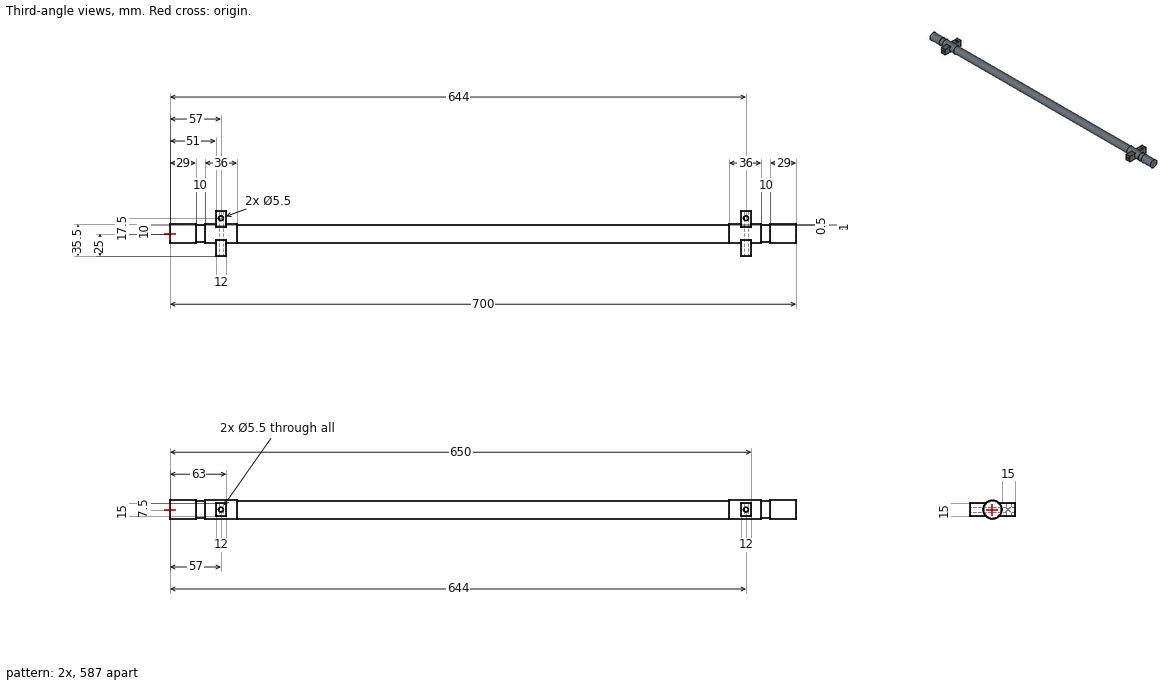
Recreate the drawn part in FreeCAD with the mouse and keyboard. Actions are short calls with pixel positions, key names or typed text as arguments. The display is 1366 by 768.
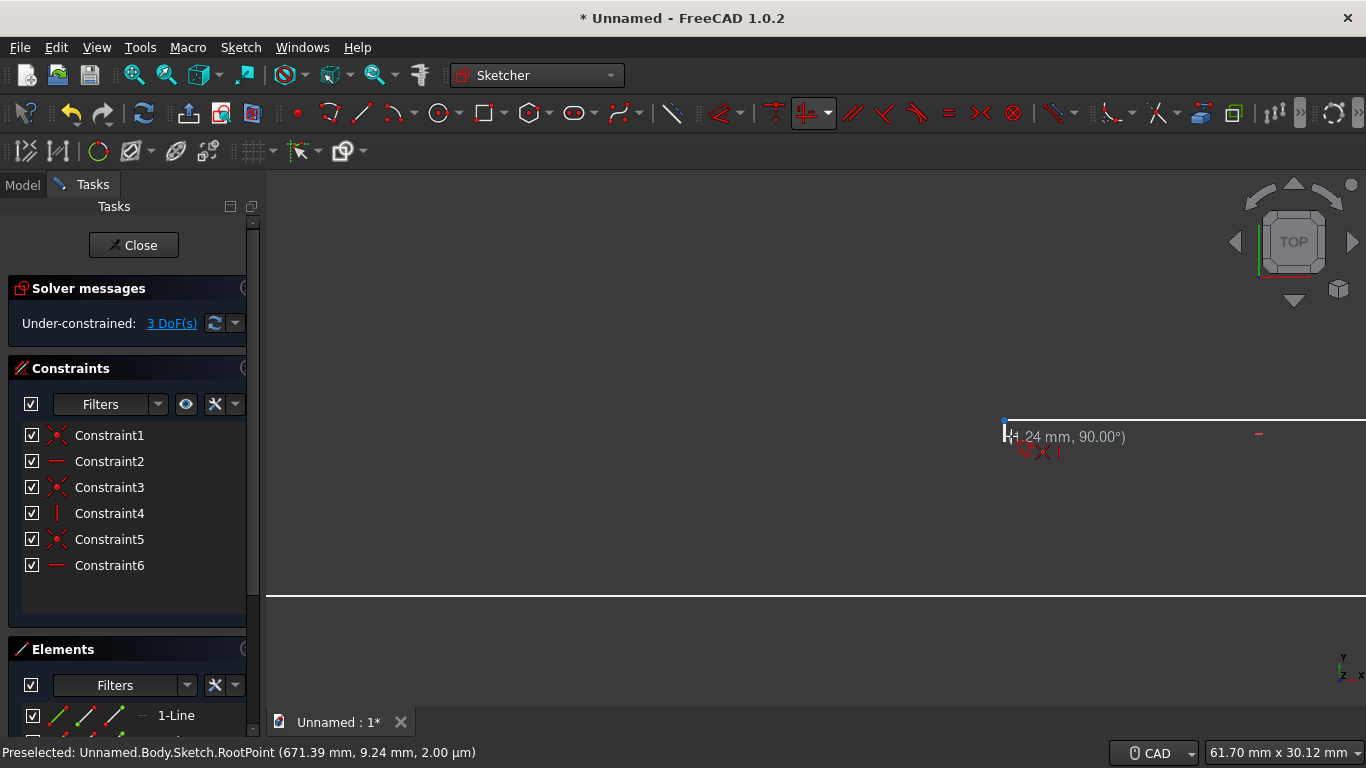
click(1004, 426)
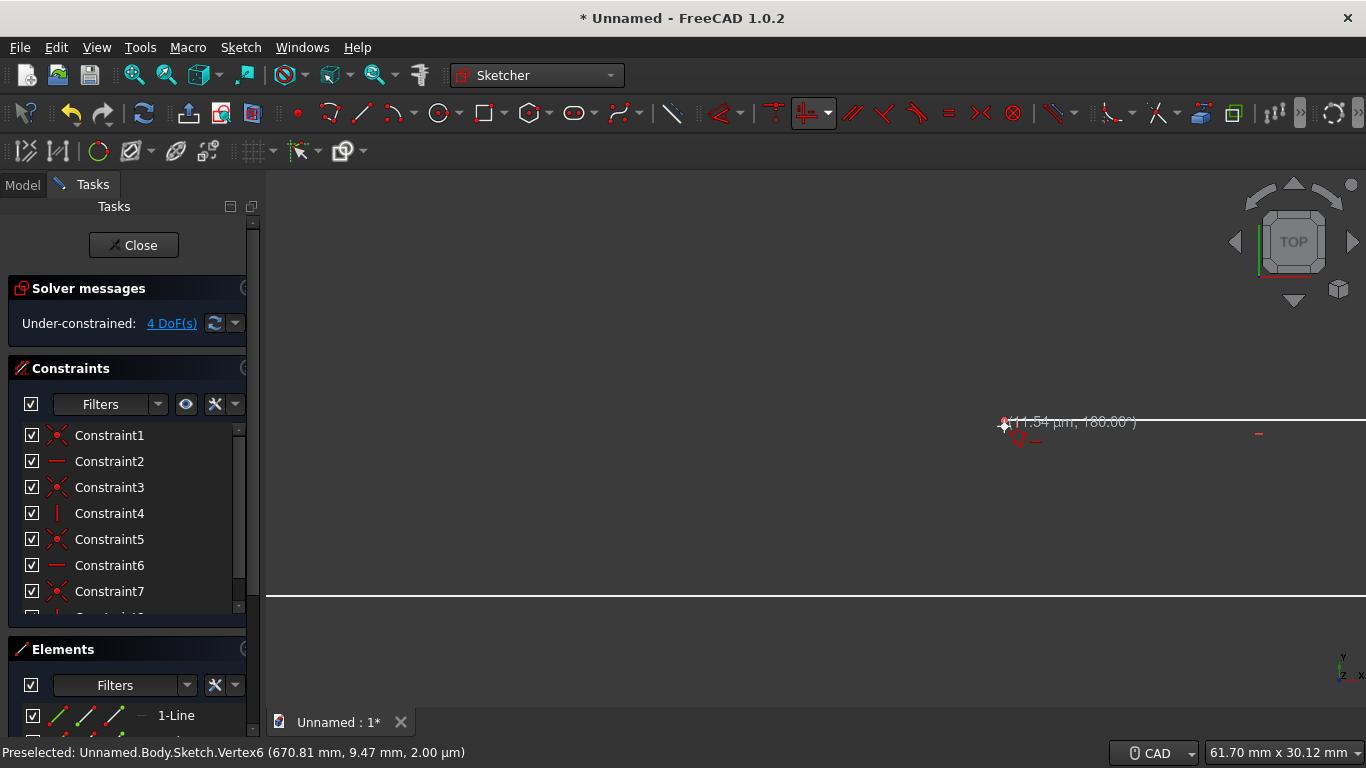
scroll(1034, 435, down, 15)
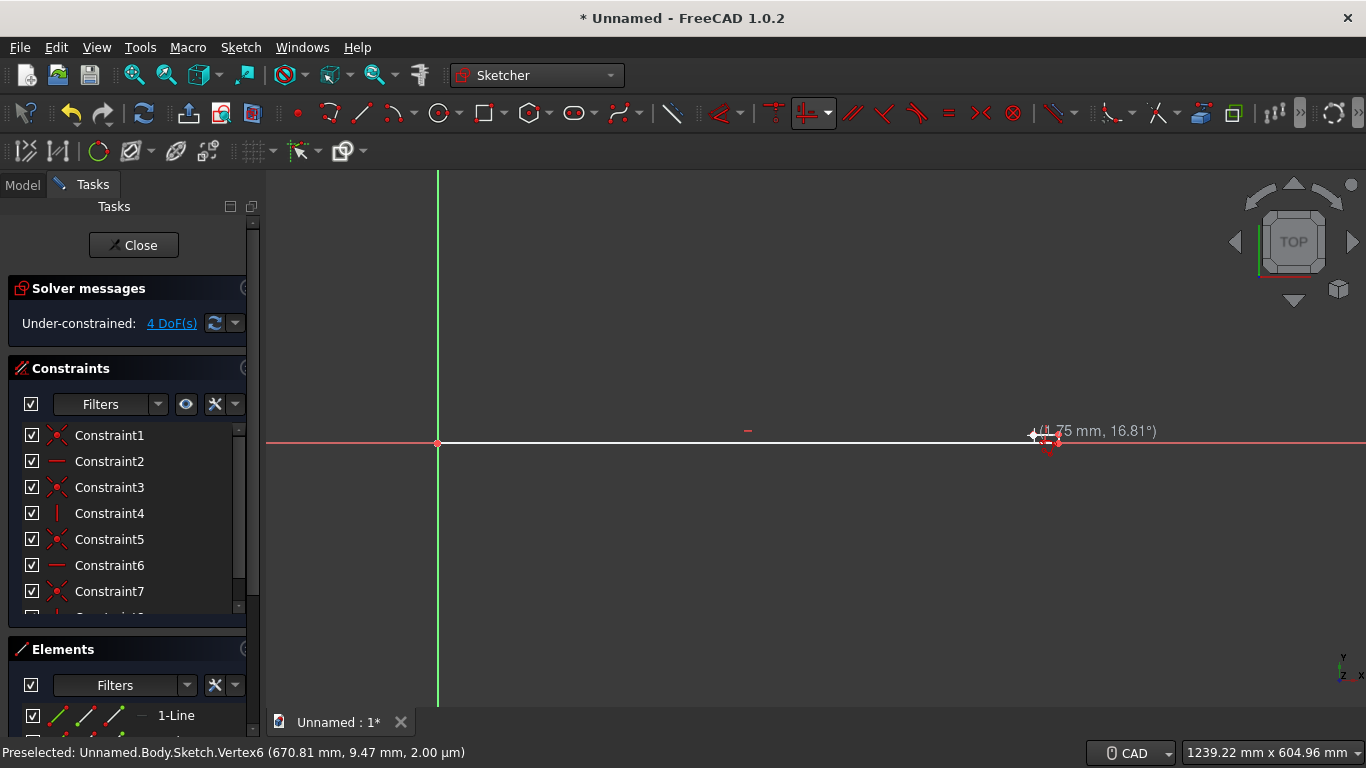
scroll(1025, 435, up, 4)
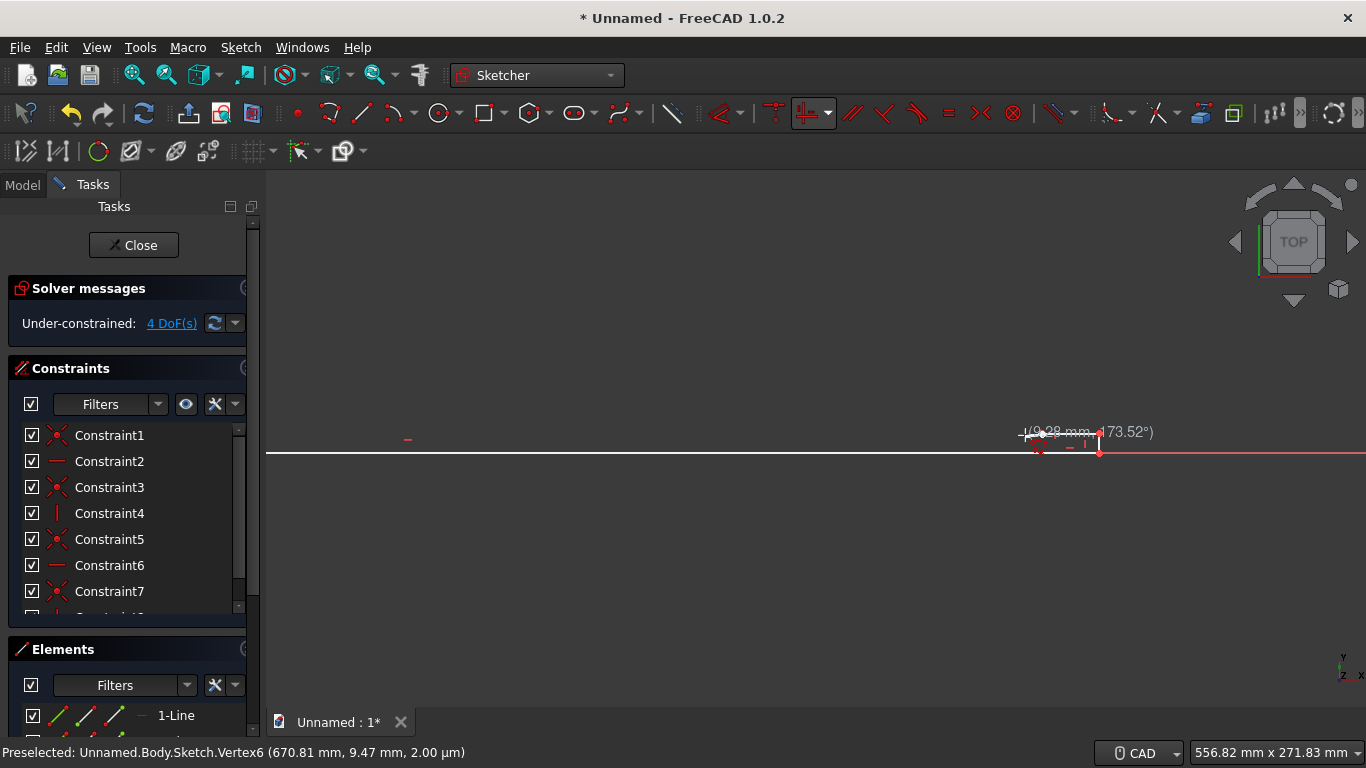
click(1023, 434)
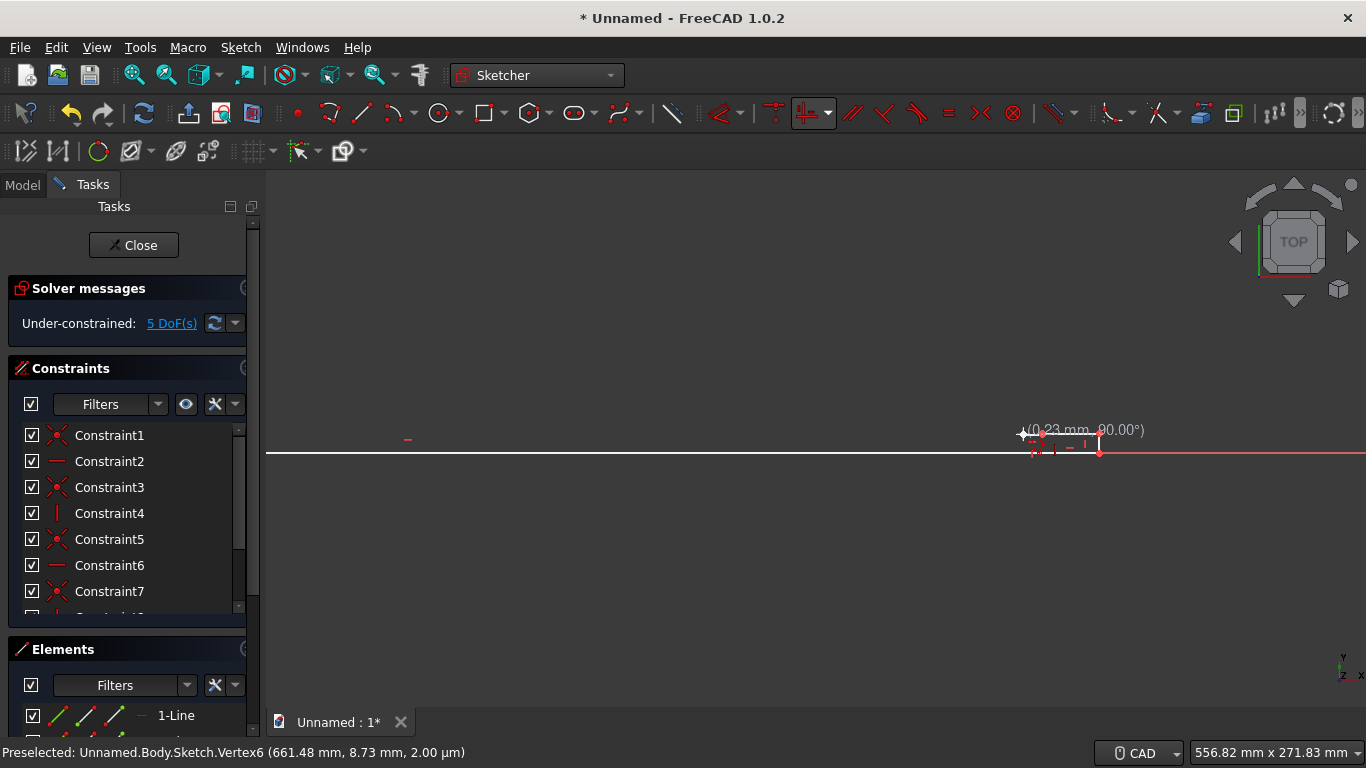
scroll(1023, 433, up, 11)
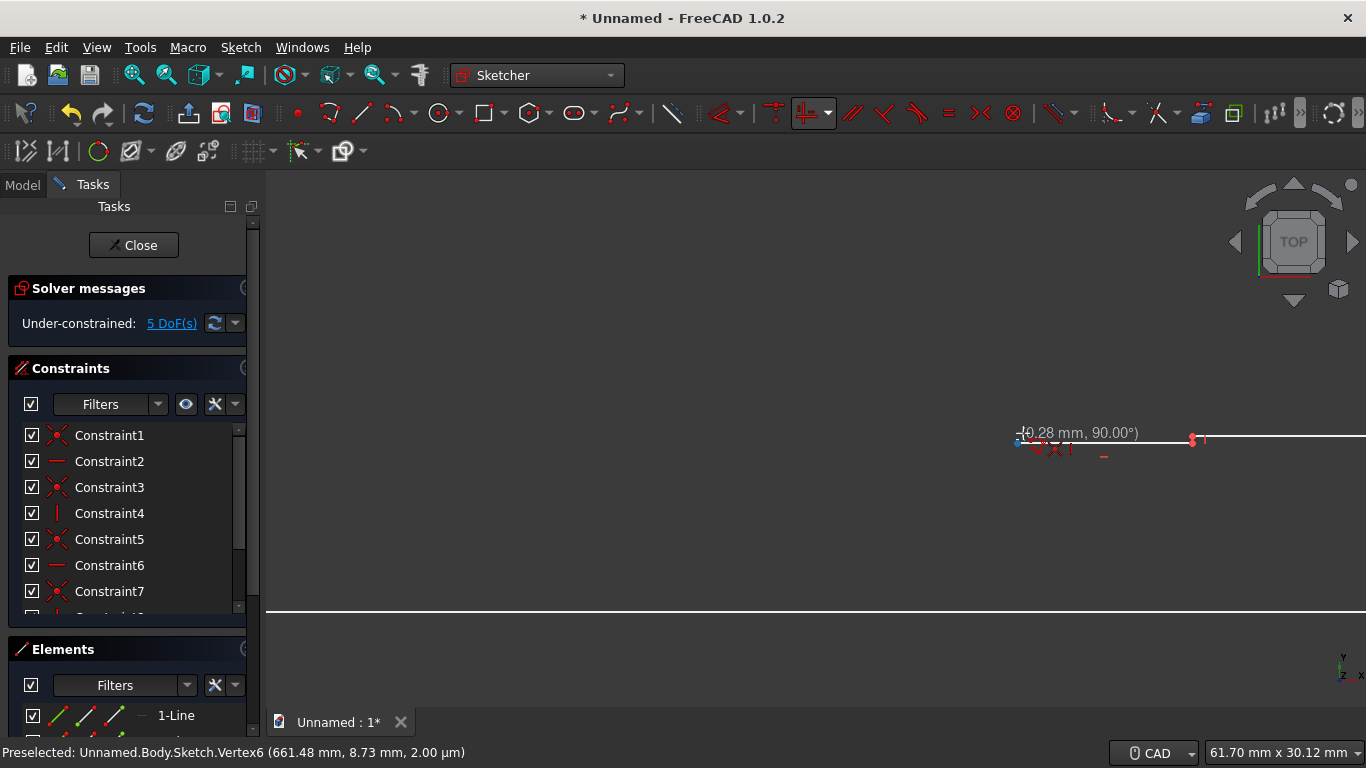
click(1017, 425)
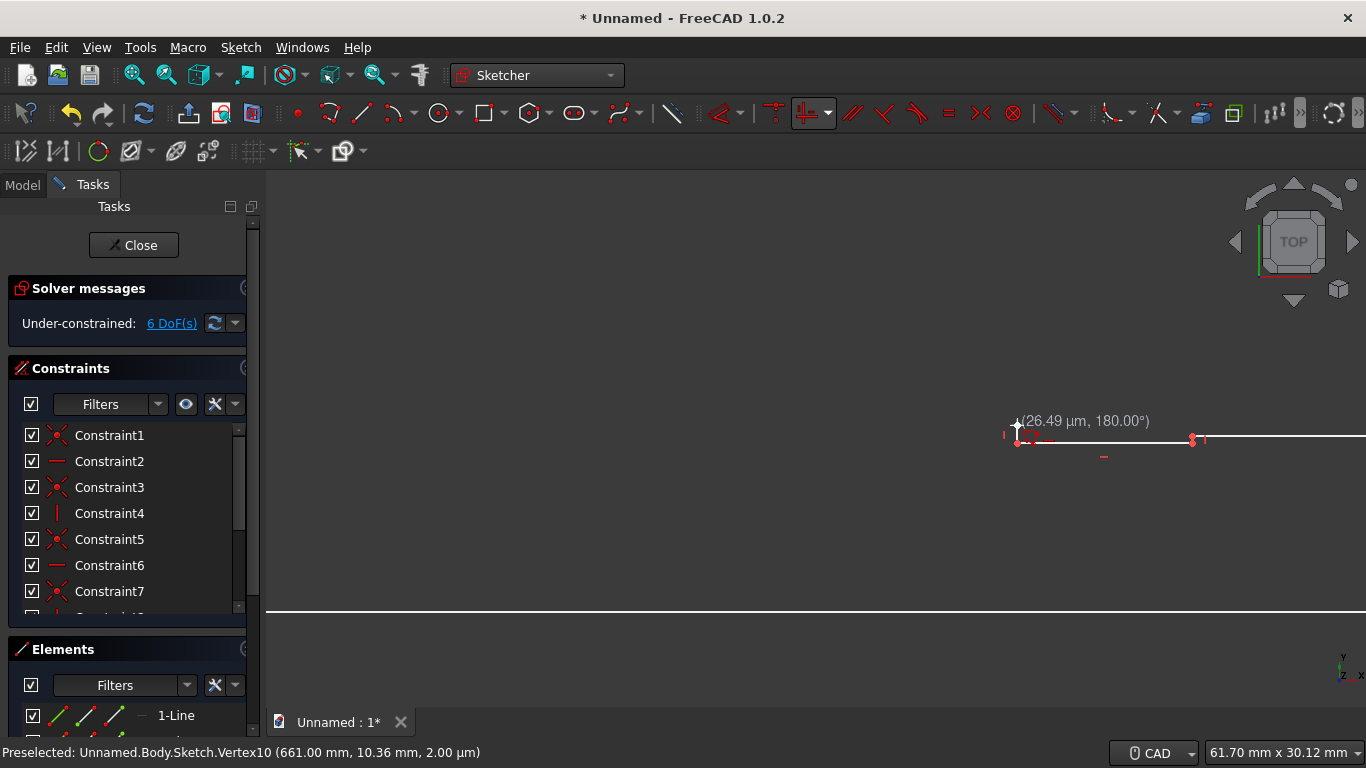
scroll(1024, 434, down, 15)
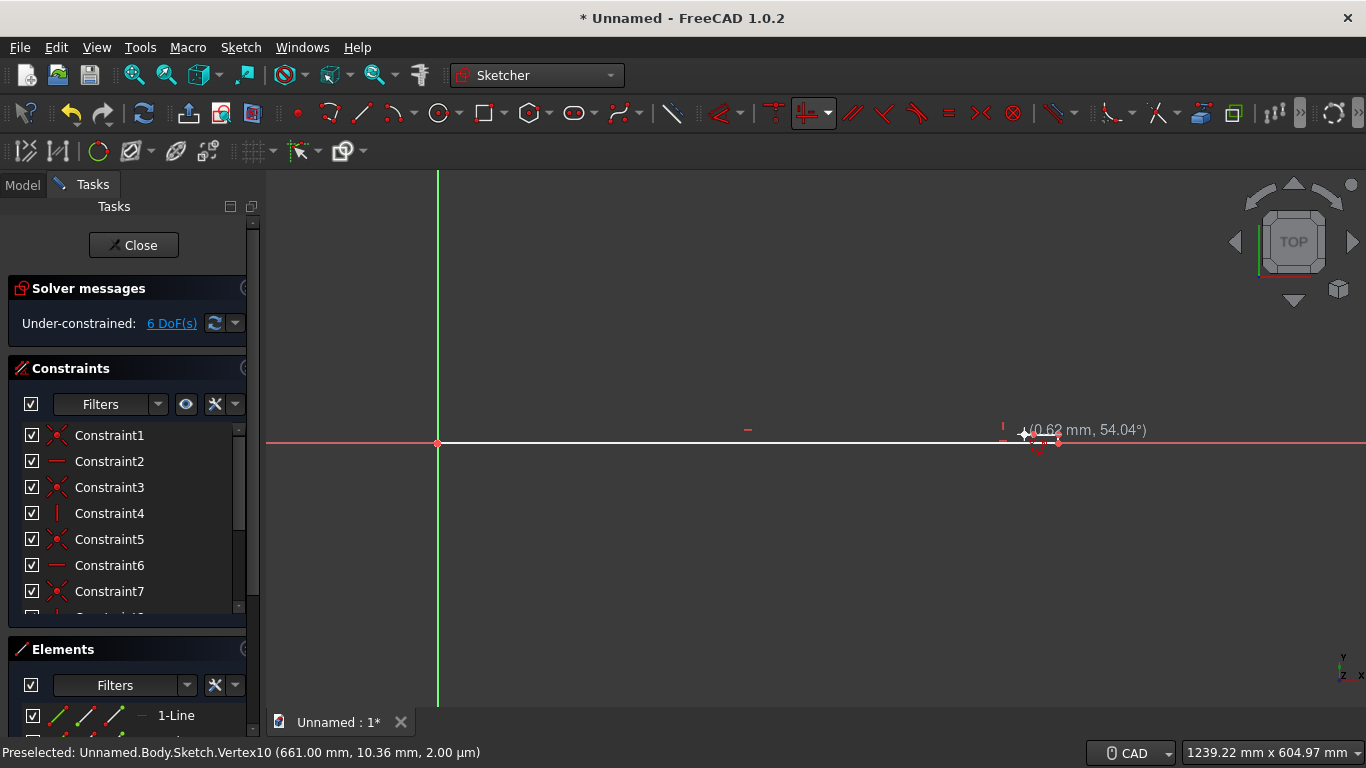
scroll(992, 434, up, 3)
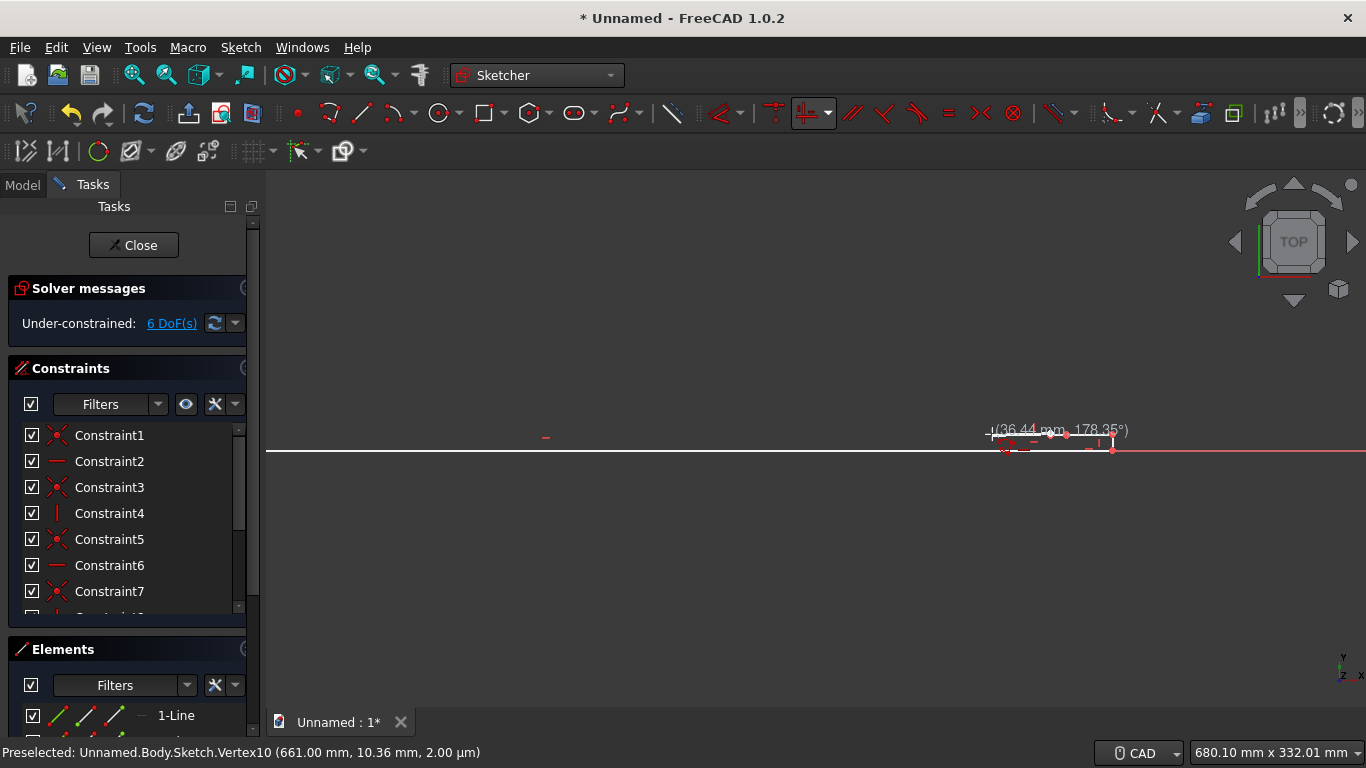
click(992, 434)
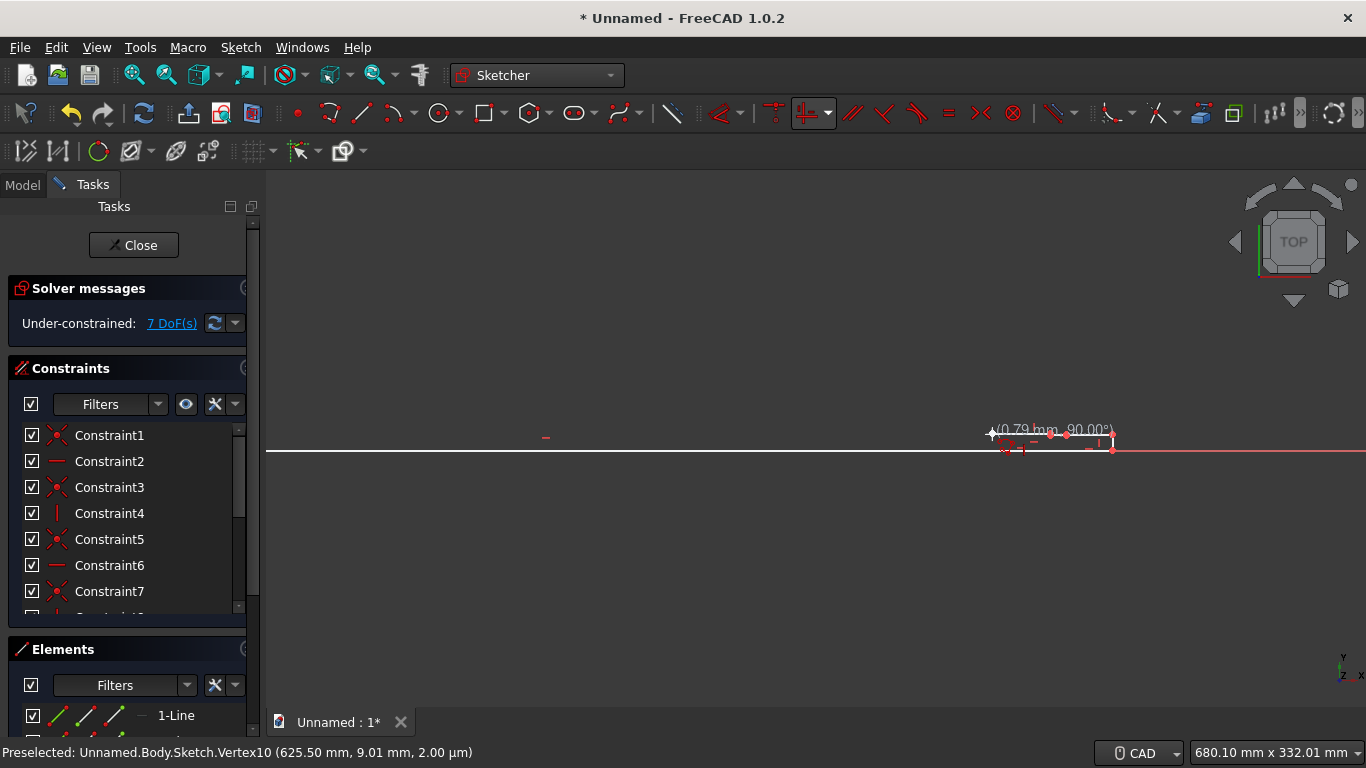
scroll(992, 434, up, 15)